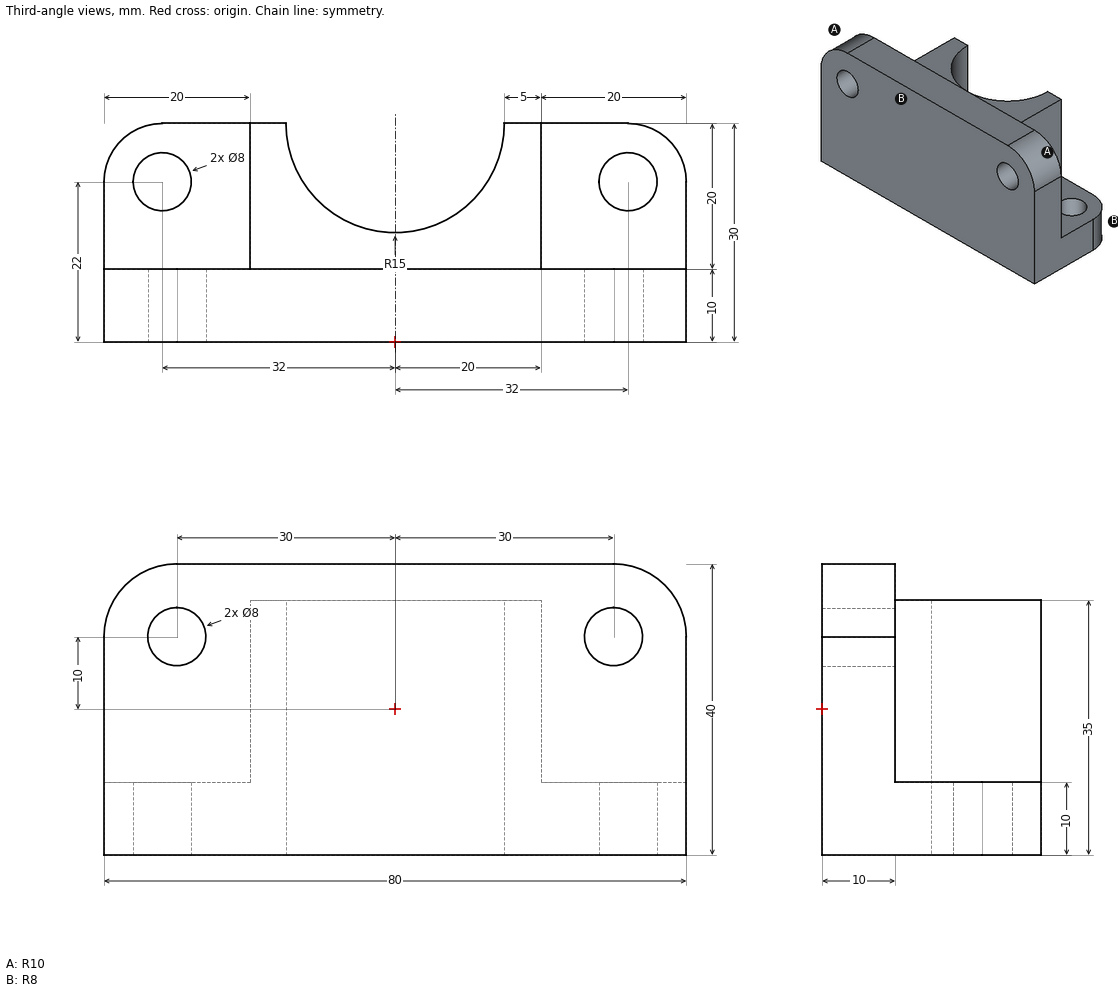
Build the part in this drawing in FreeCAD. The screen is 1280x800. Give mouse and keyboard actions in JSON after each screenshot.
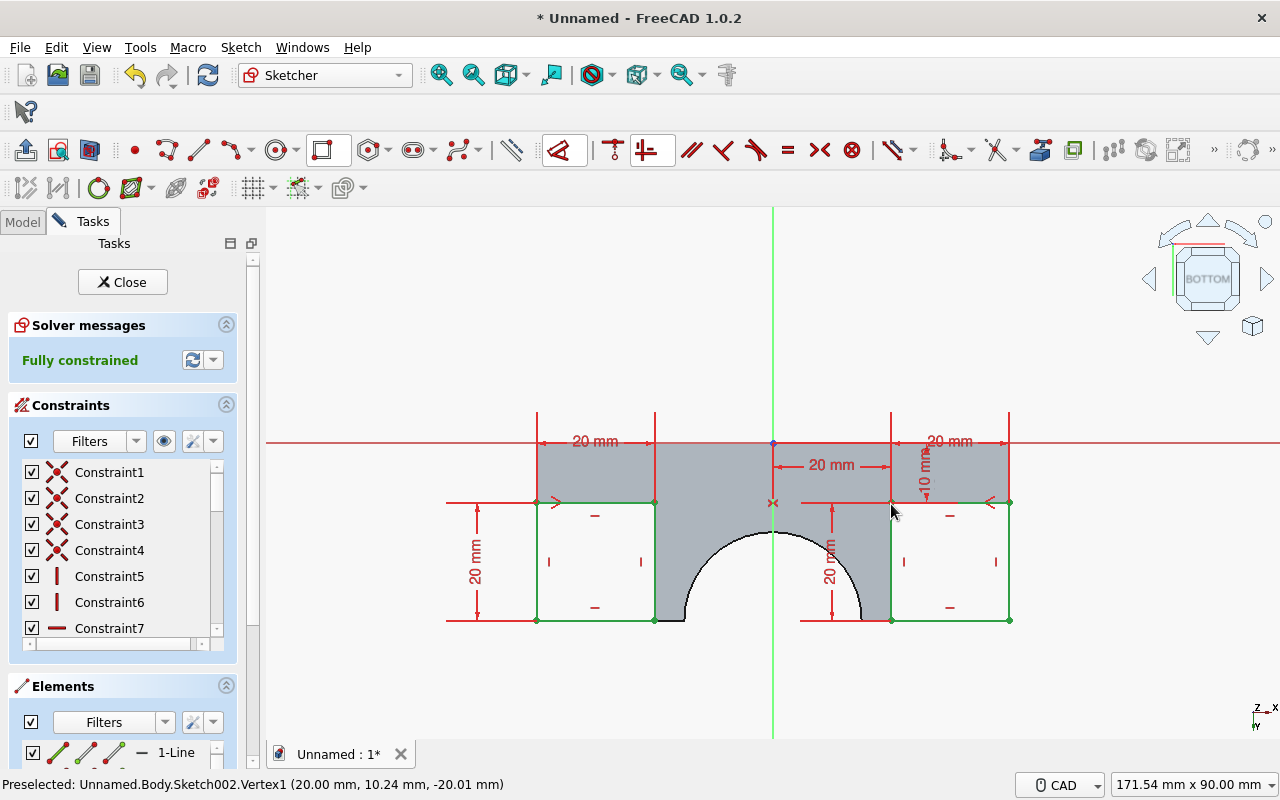
{"action": "left_click", "coordinate": [123, 282]}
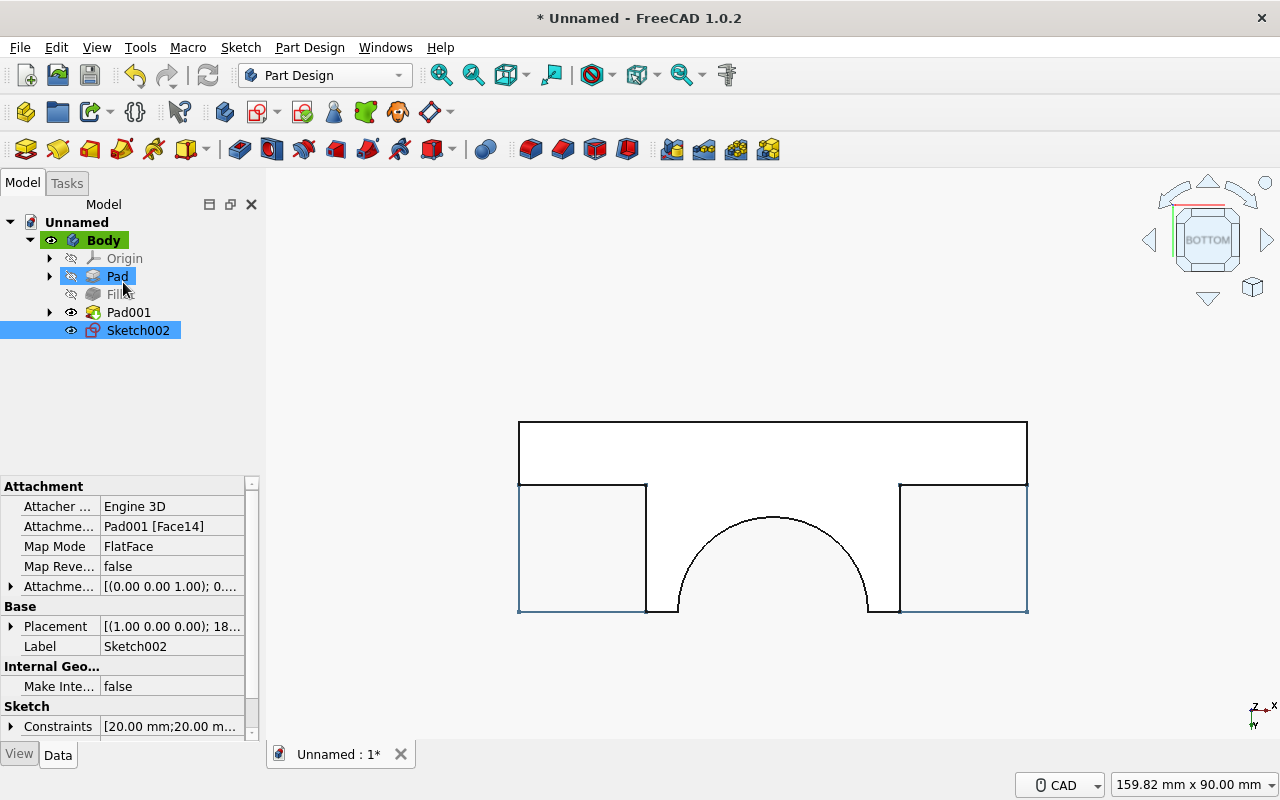
{"action": "left_click", "coordinate": [26, 150]}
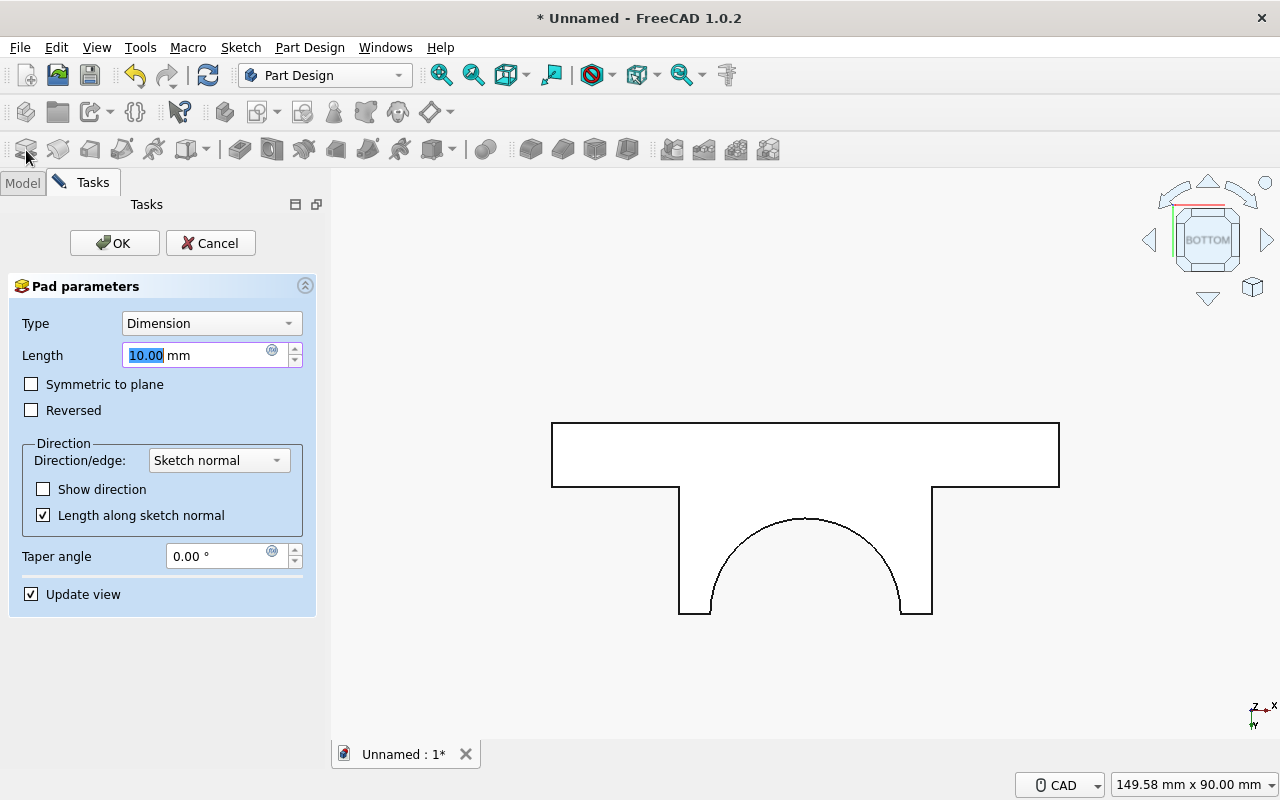
{"action": "type", "text": "10"}
{"action": "key", "text": "Tab"}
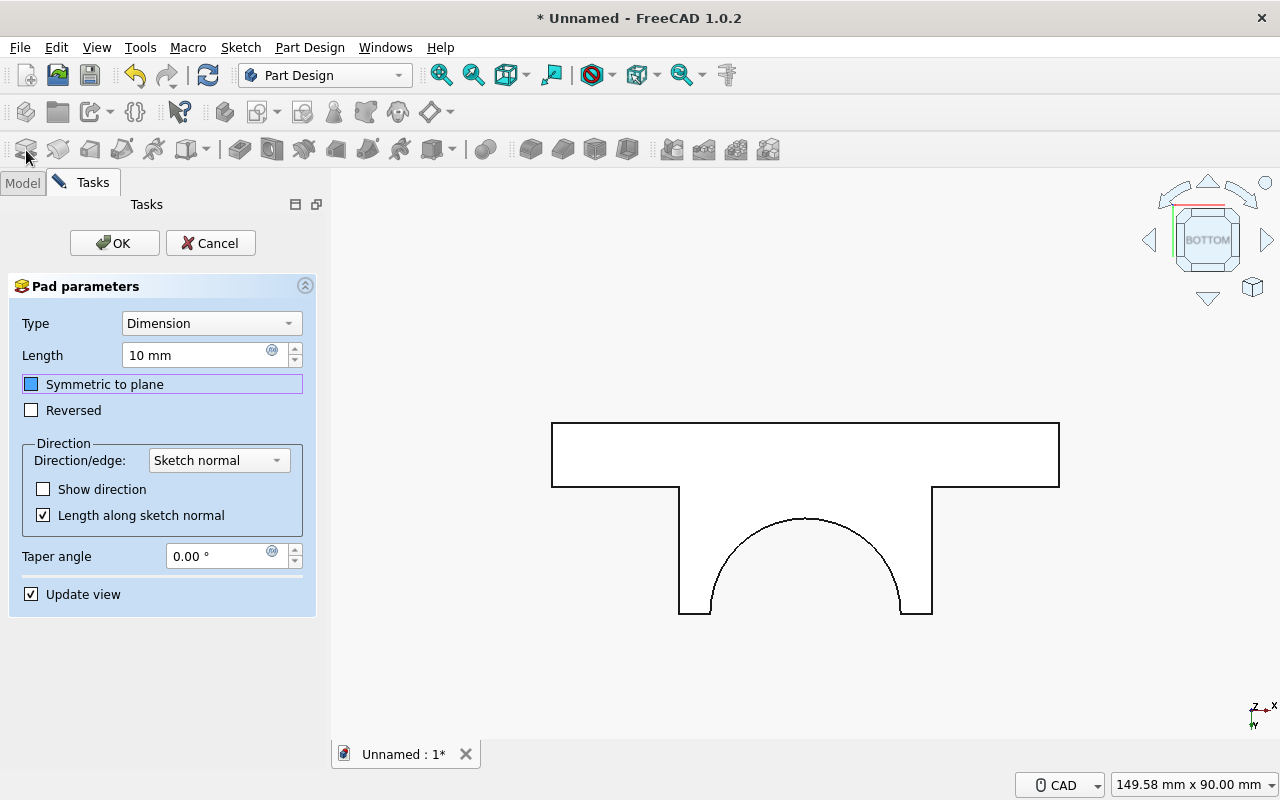
{"action": "left_click", "coordinate": [30, 410]}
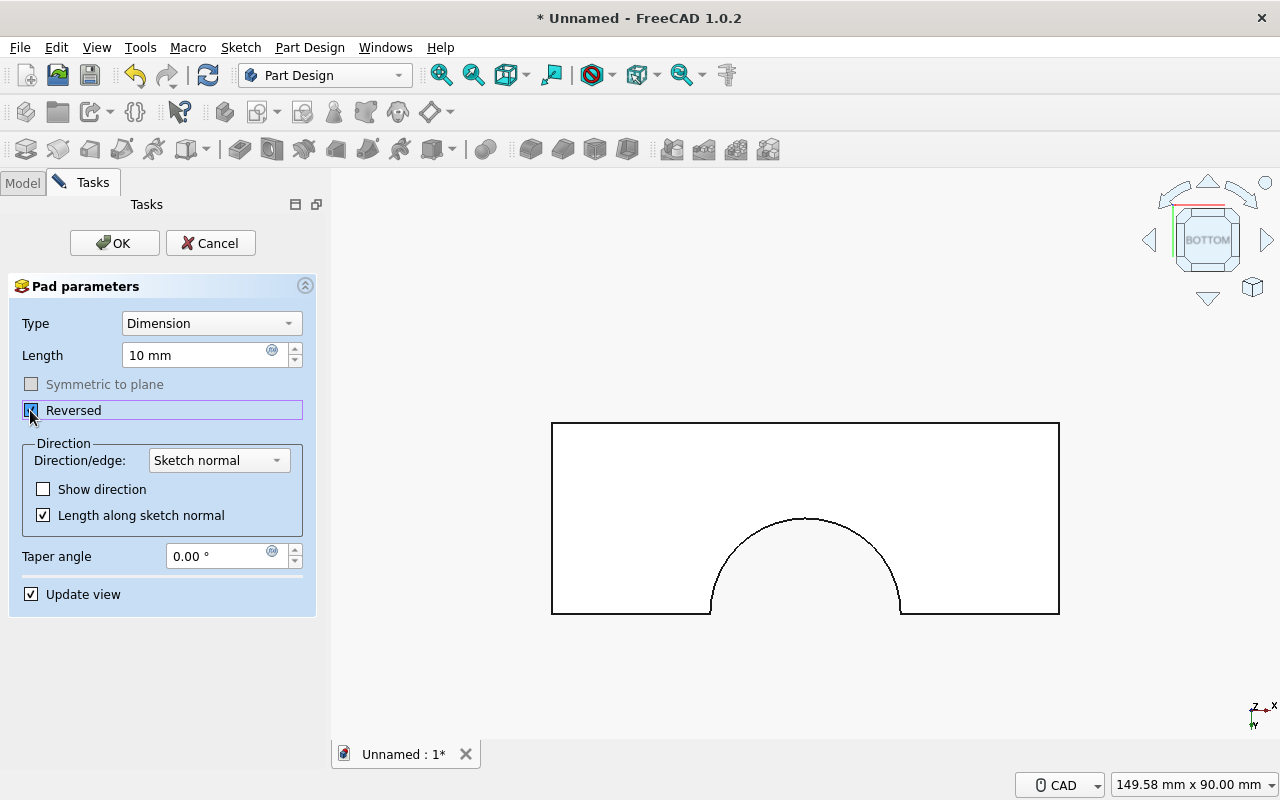
{"action": "left_click", "coordinate": [115, 243]}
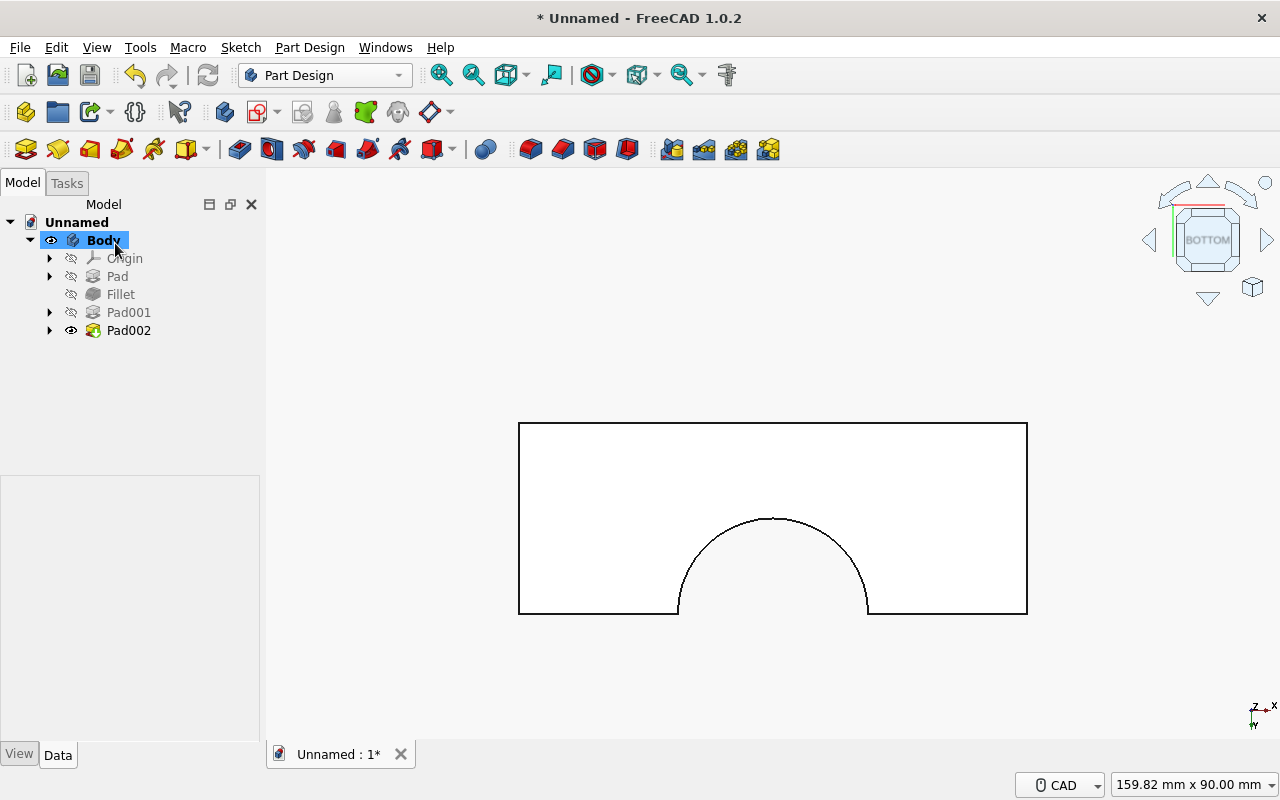
{"action": "key", "text": "0"}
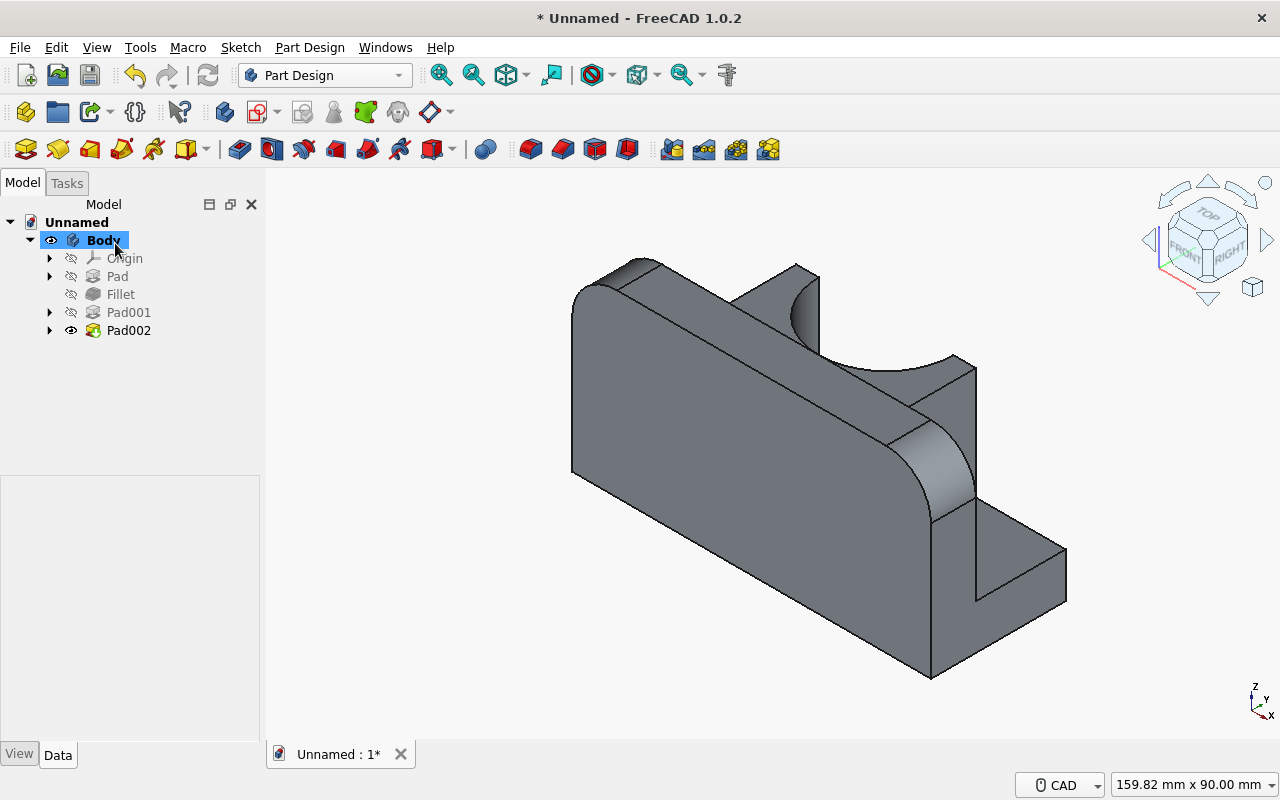
{"action": "key", "text": "2"}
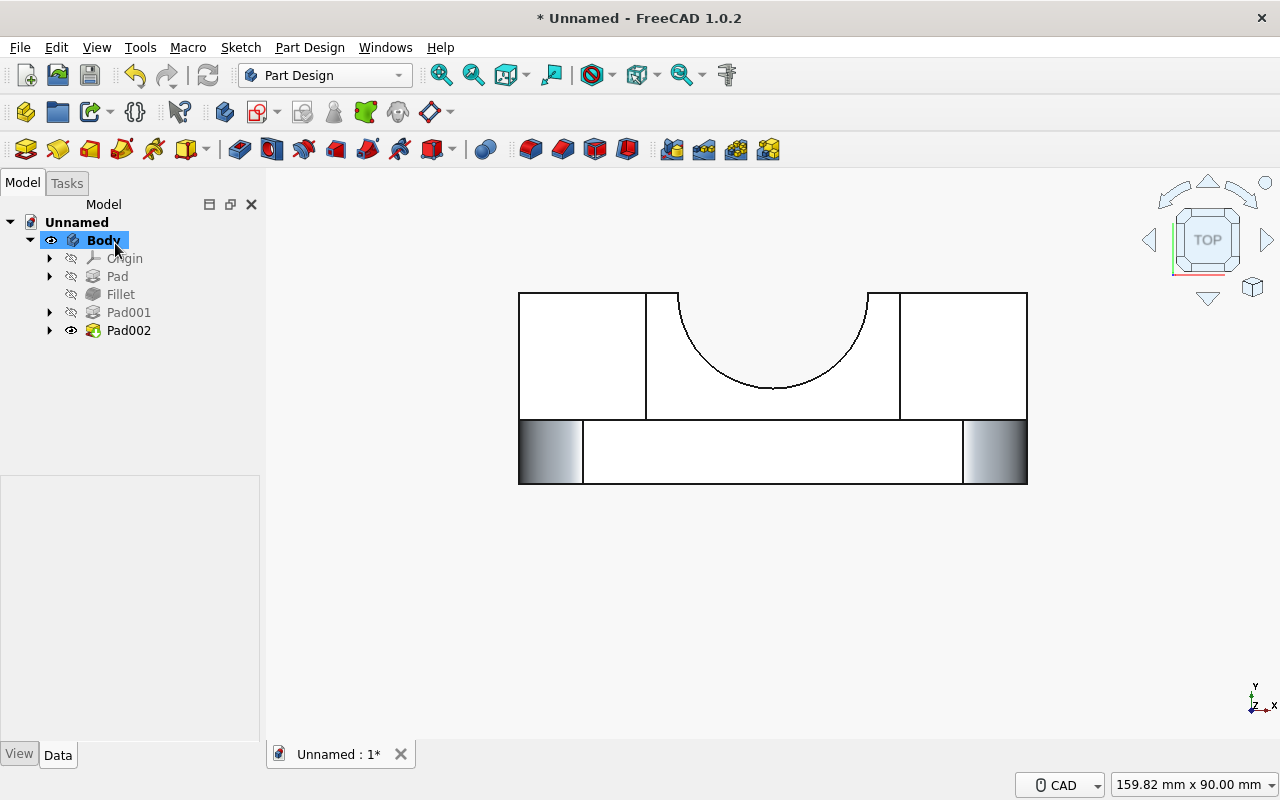
{"action": "key", "text": "1"}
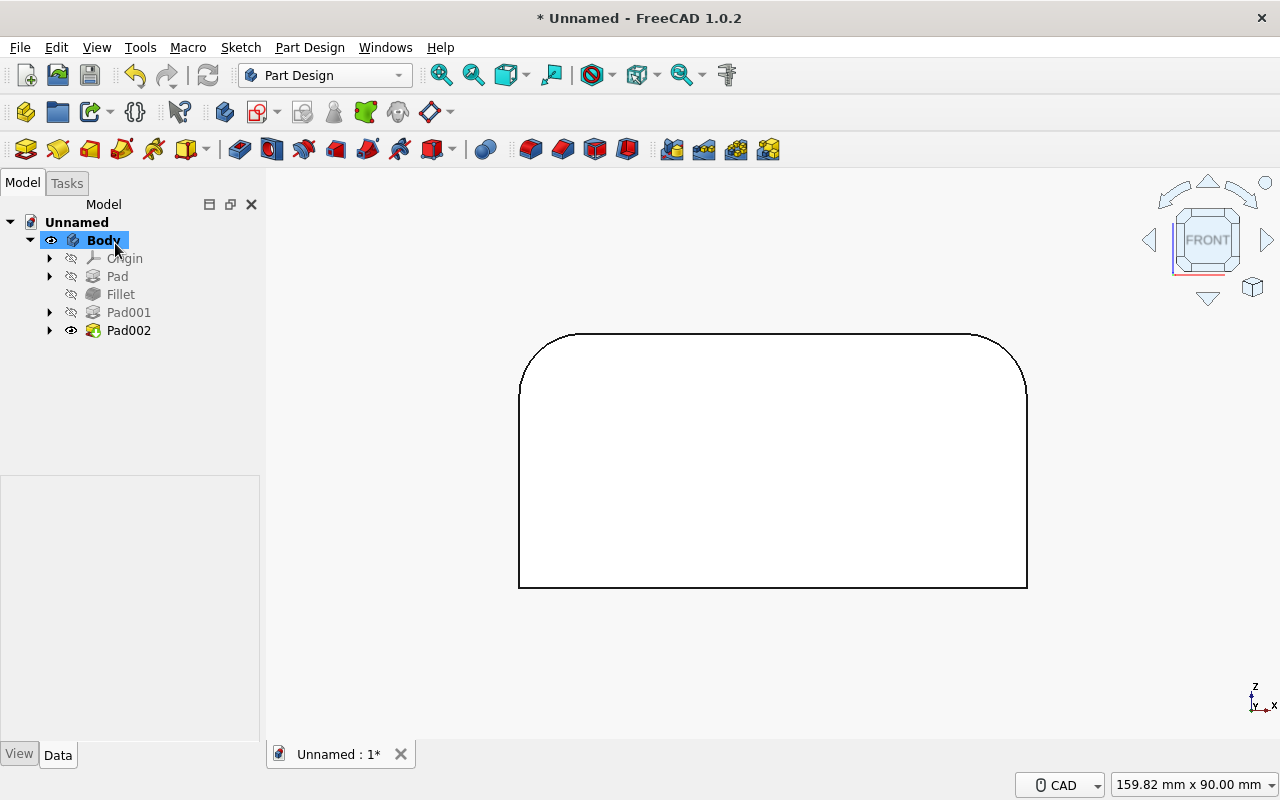
{"action": "key", "text": "3"}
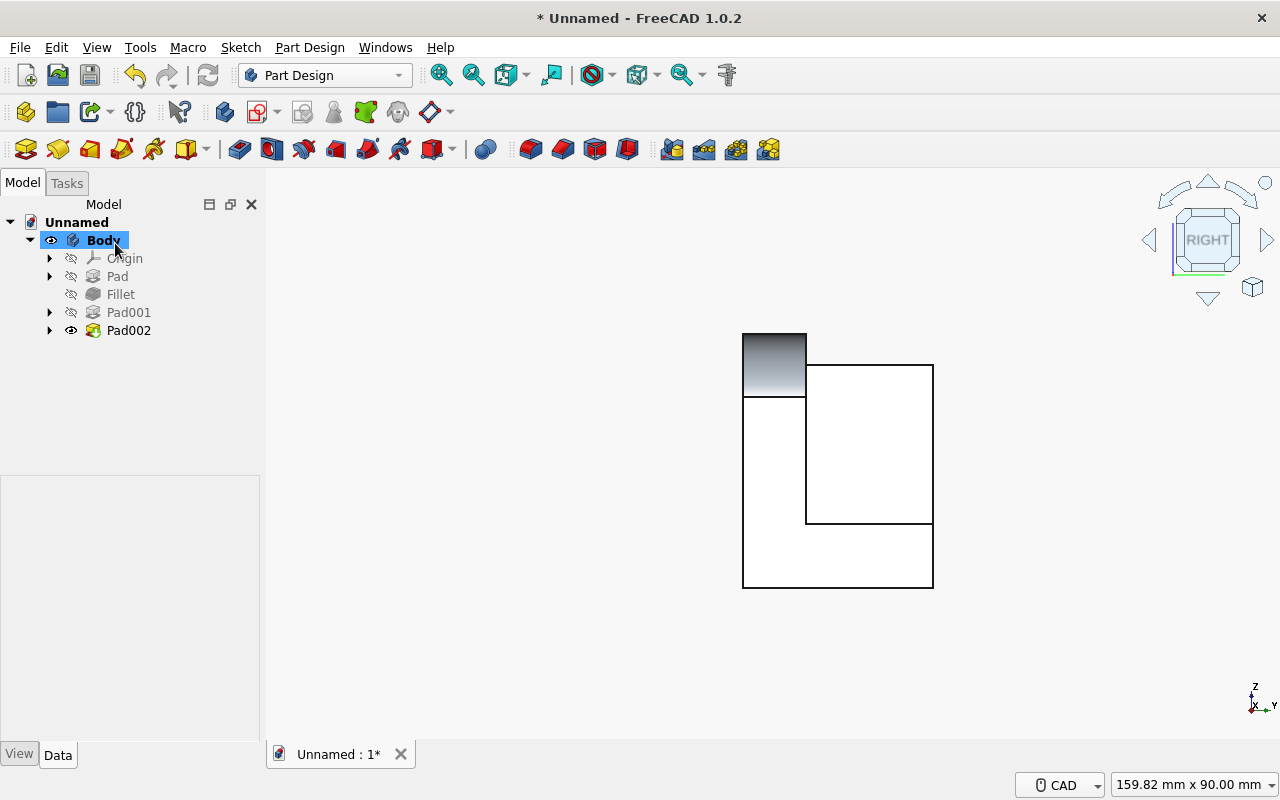
{"action": "left_click", "coordinate": [442, 76]}